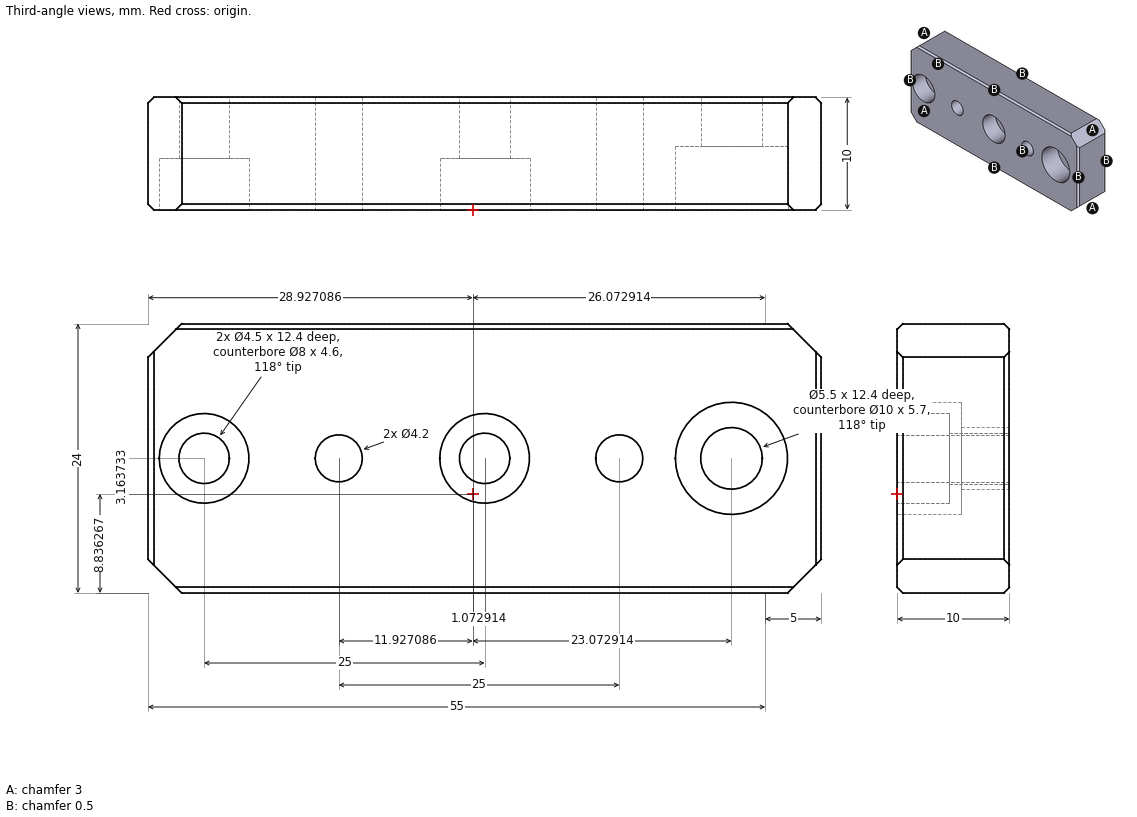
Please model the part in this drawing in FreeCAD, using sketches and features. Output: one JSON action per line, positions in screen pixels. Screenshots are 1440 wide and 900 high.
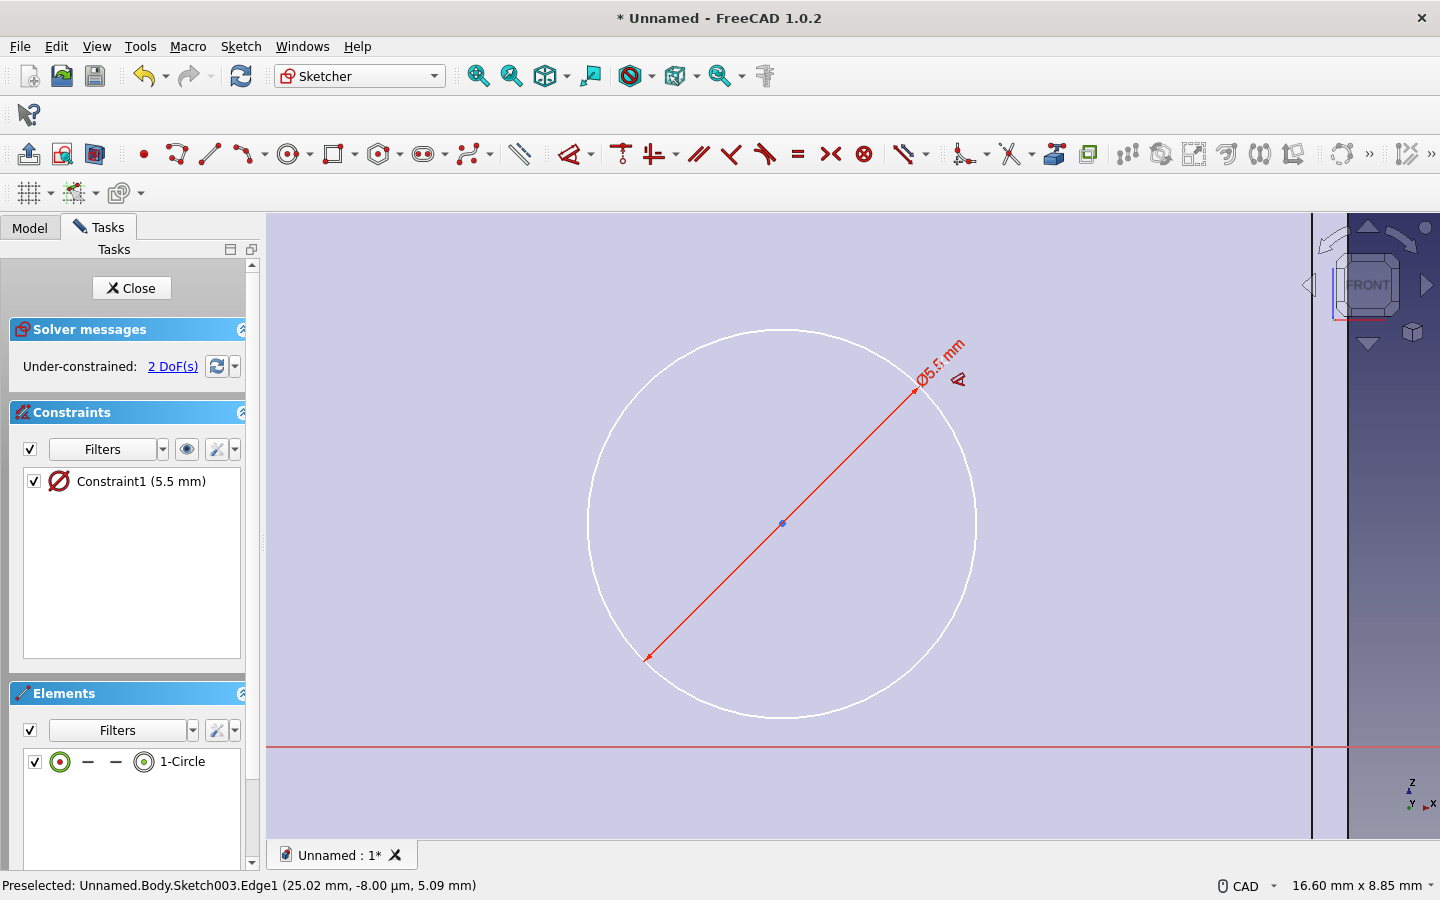
{"action": "left_click", "coordinate": [782, 524]}
{"action": "left_click", "coordinate": [816, 635]}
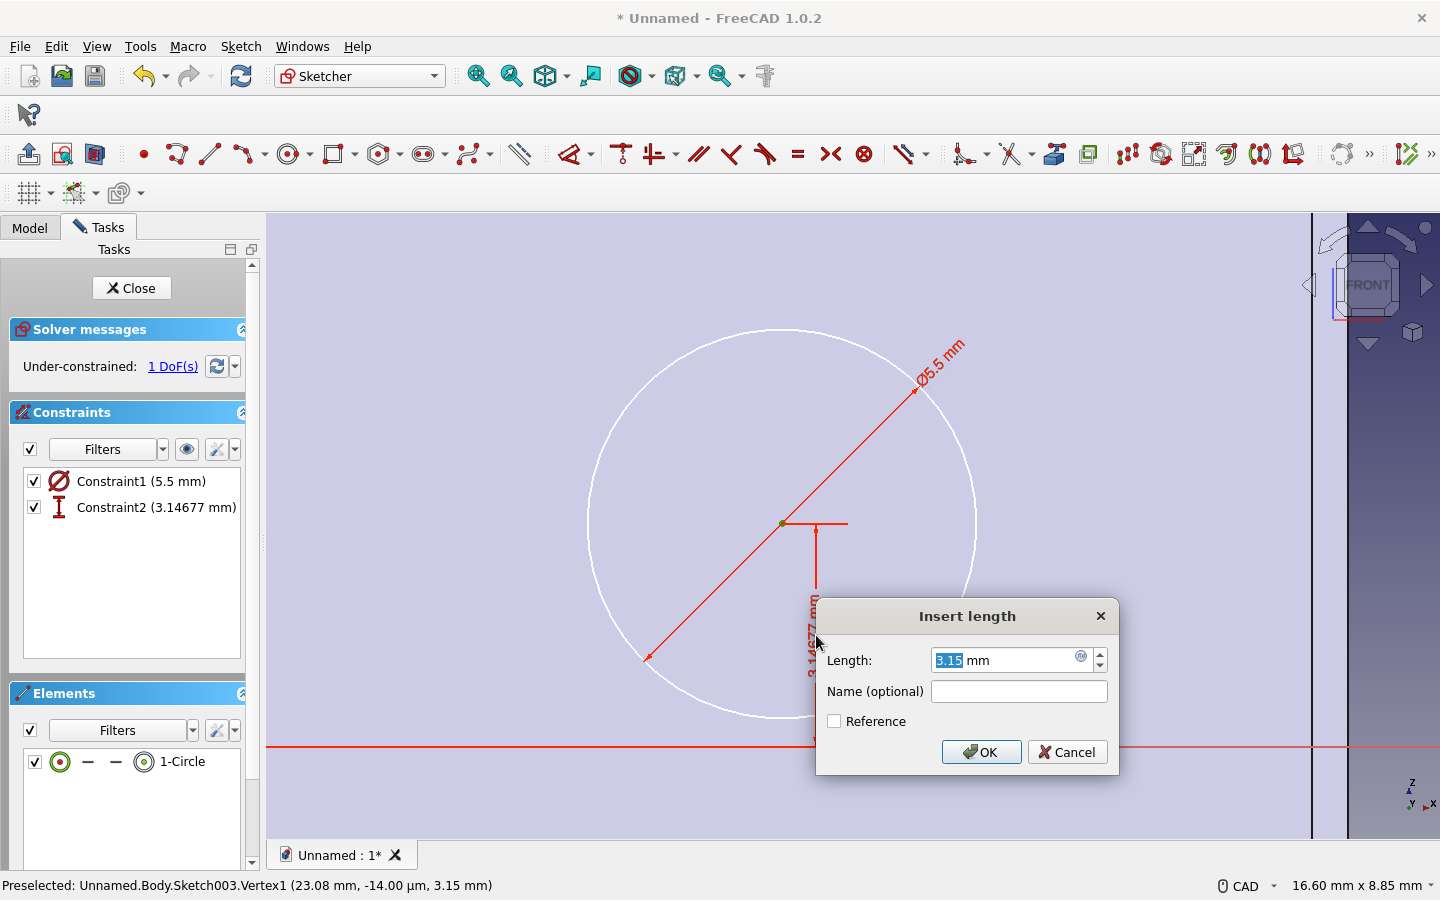
{"action": "type", "text": "3.163733"}
{"action": "key", "text": "Return"}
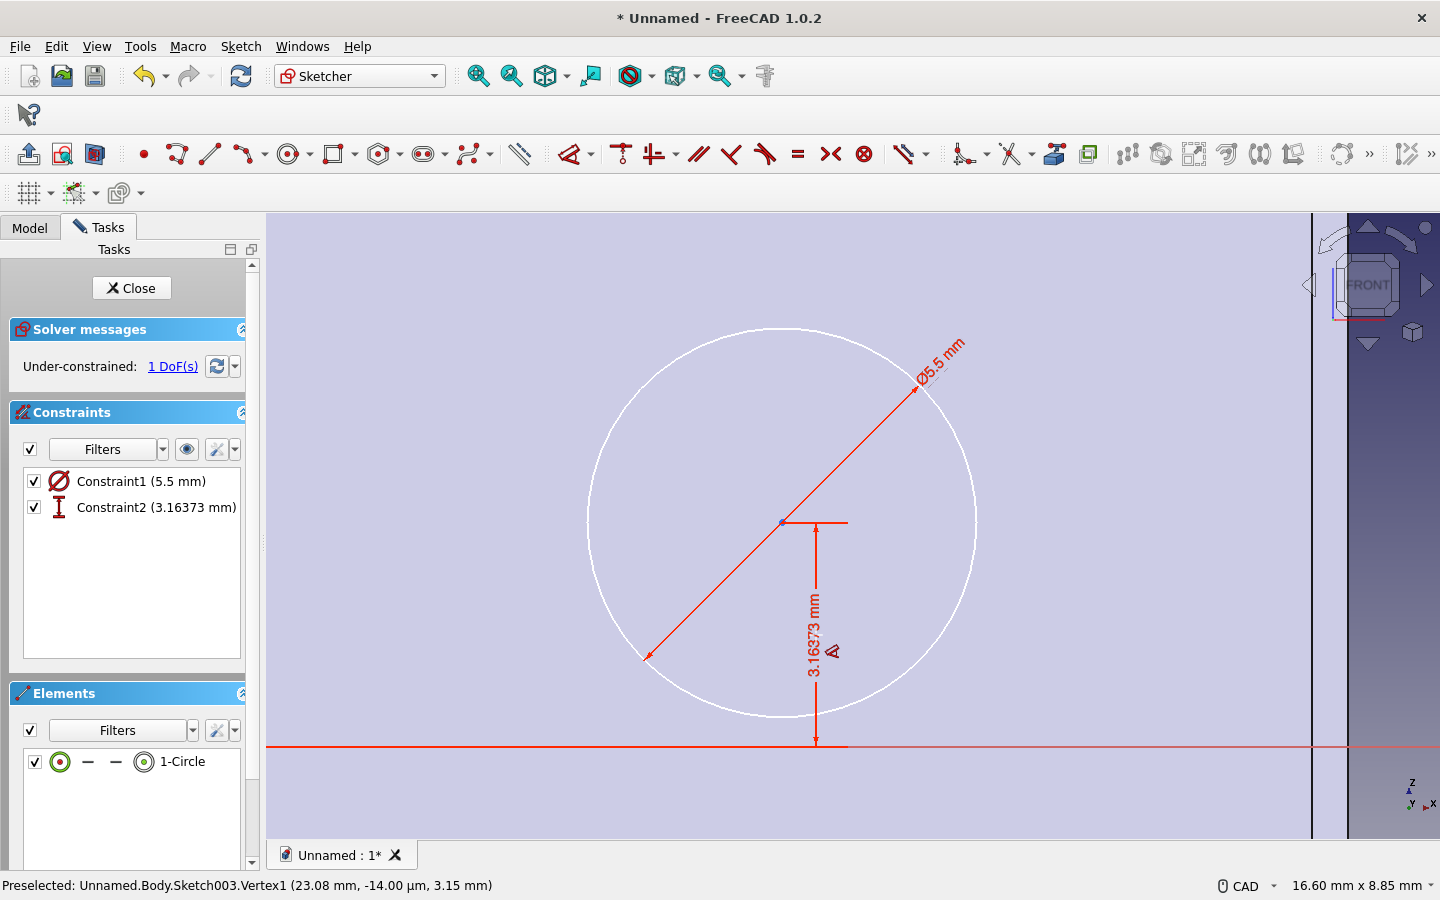
{"action": "left_click", "coordinate": [782, 523]}
{"action": "left_click", "coordinate": [538, 781]}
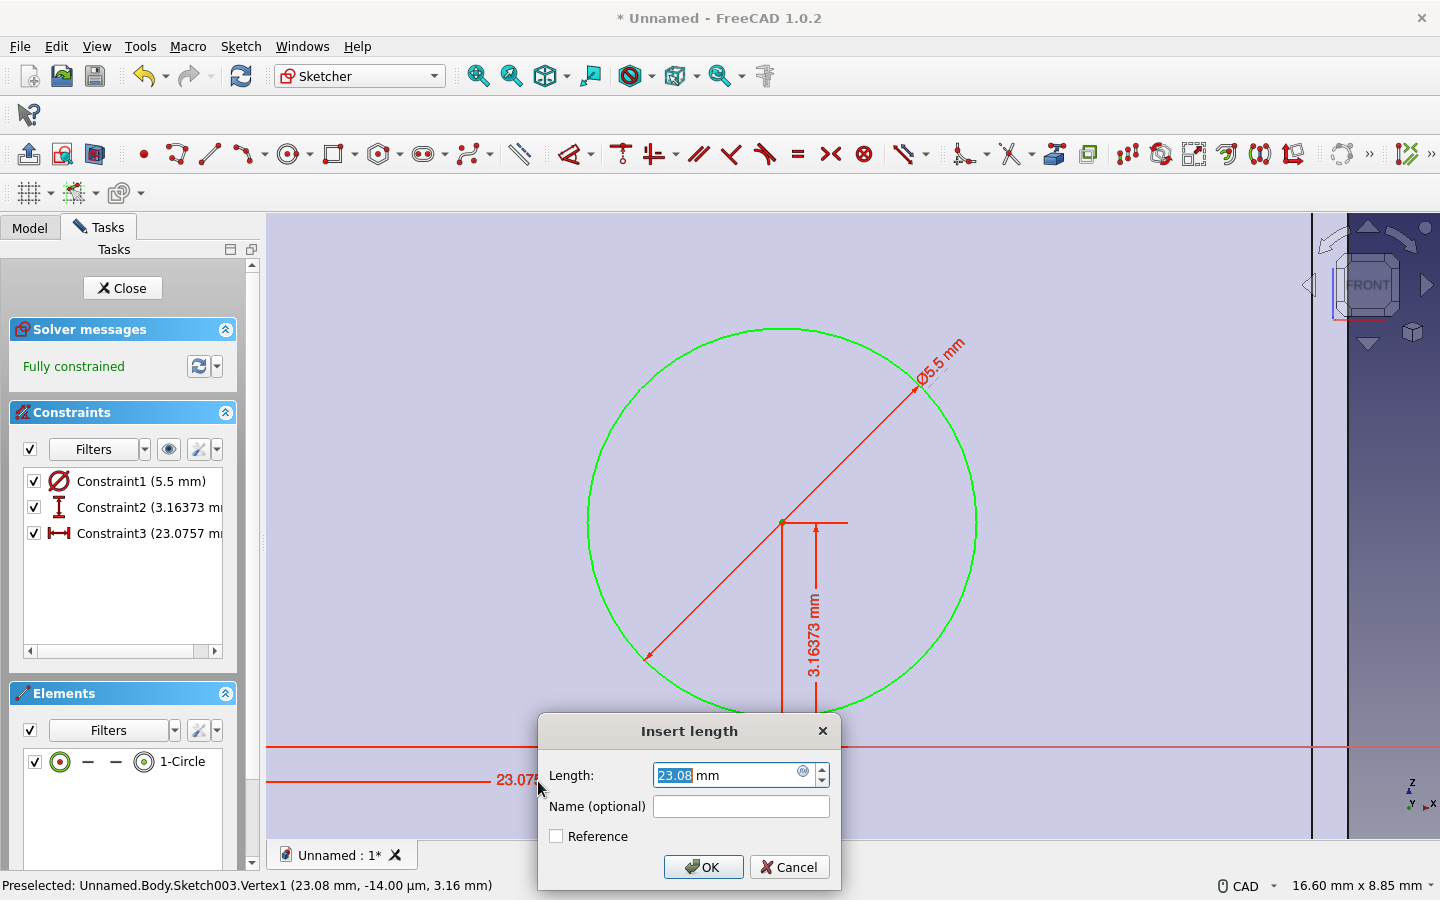
{"action": "type", "text": "23.072914"}
{"action": "key", "text": "Return"}
{"action": "key", "text": "Escape"}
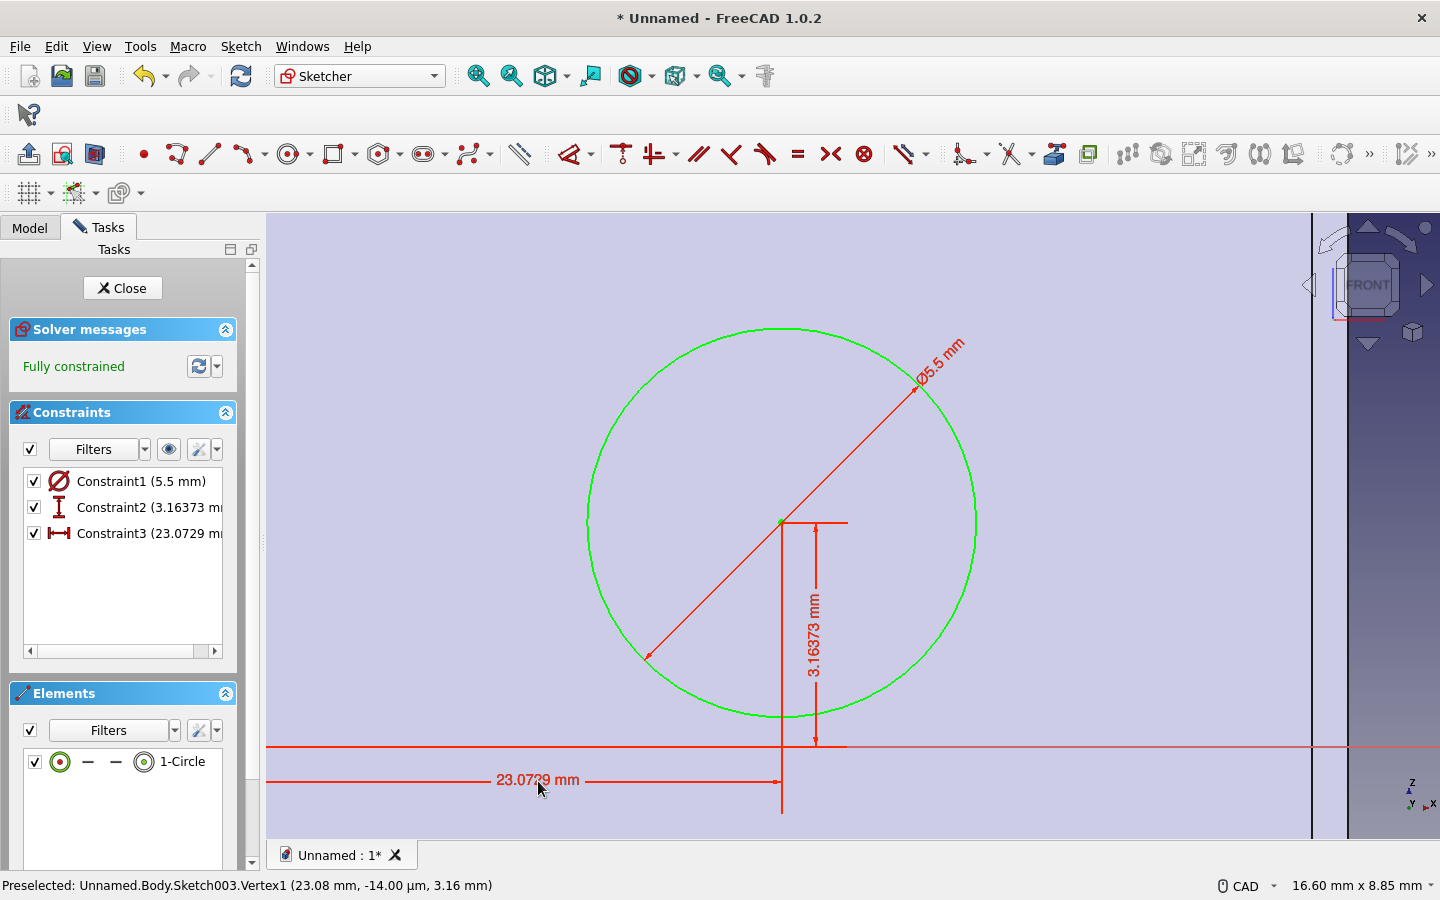
{"action": "left_click", "coordinate": [123, 288]}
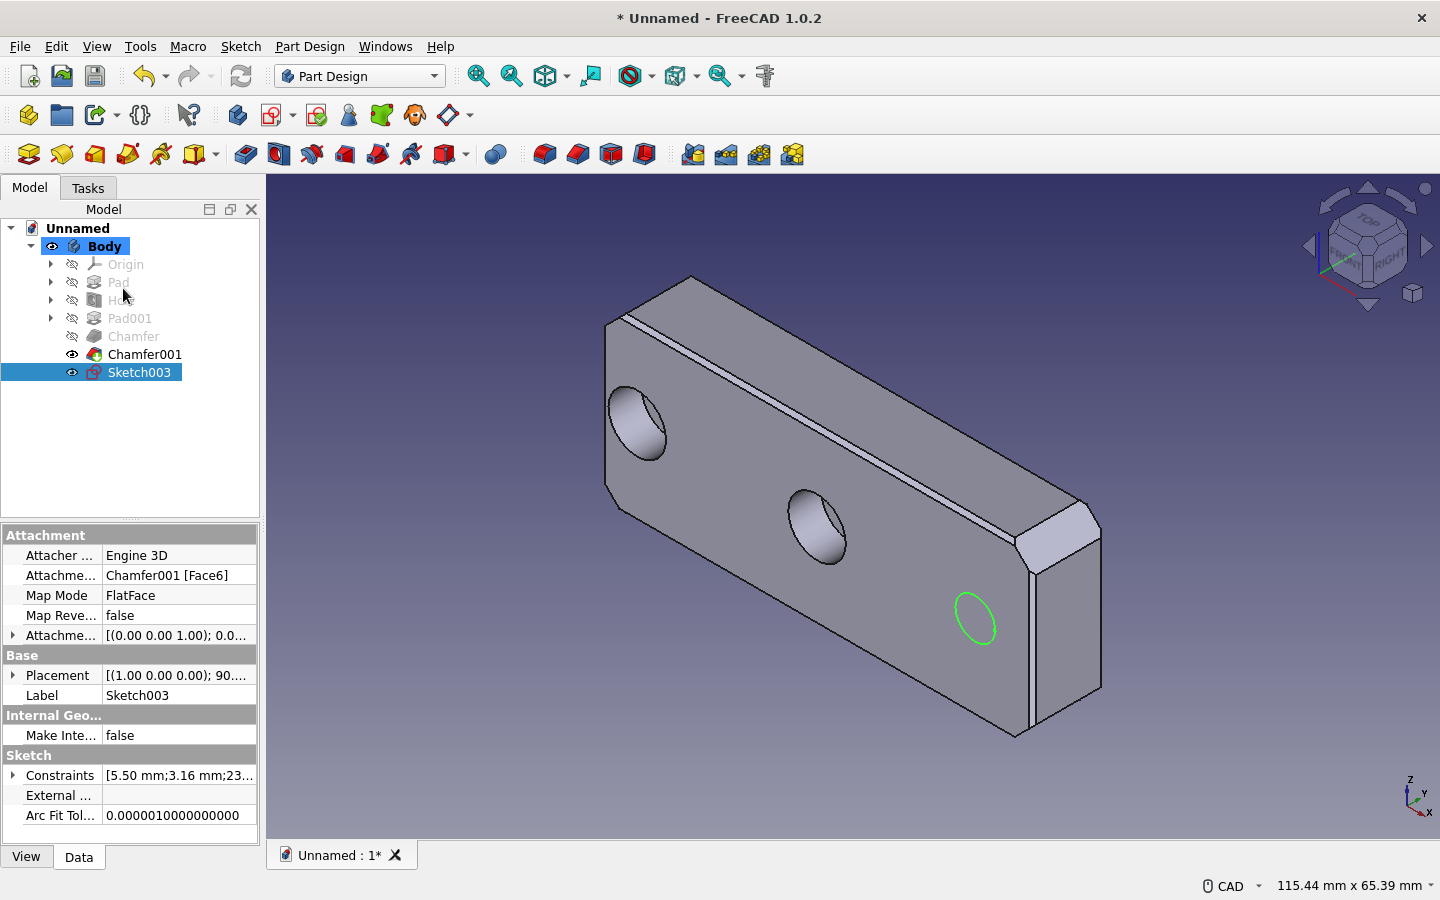
{"action": "left_click", "coordinate": [279, 154]}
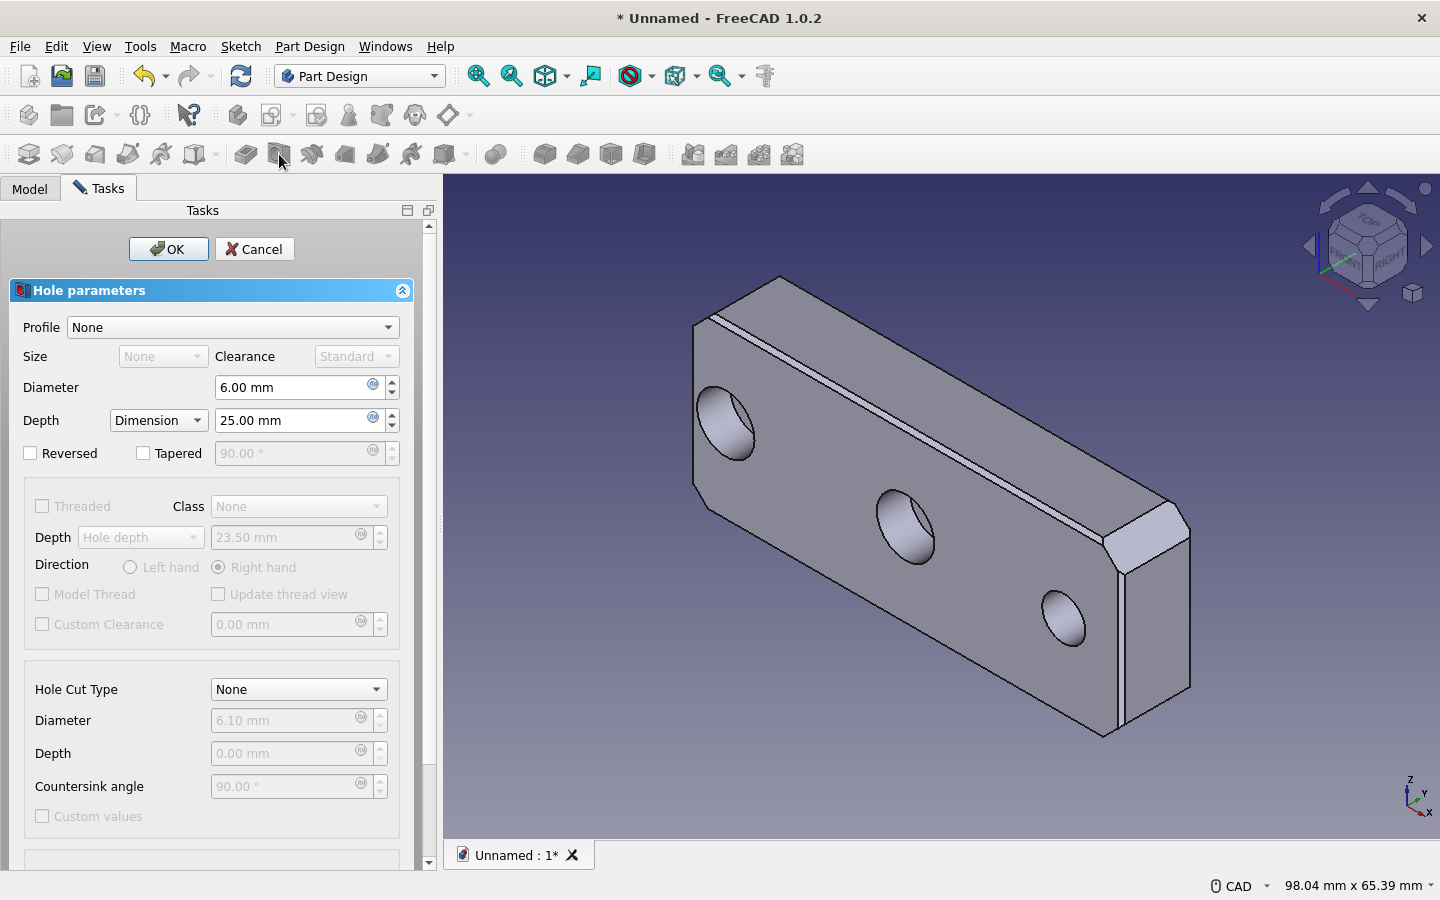
{"action": "triple_click", "coordinate": [300, 388]}